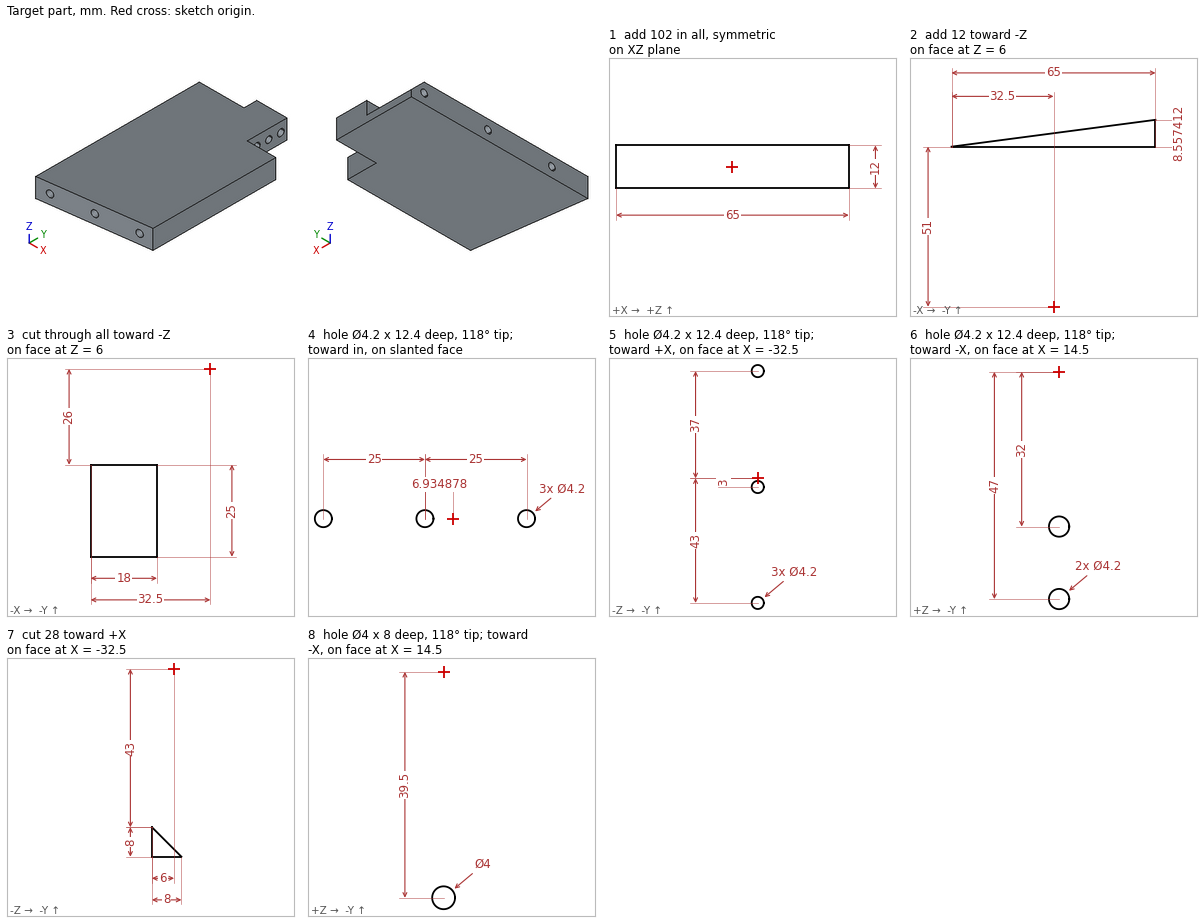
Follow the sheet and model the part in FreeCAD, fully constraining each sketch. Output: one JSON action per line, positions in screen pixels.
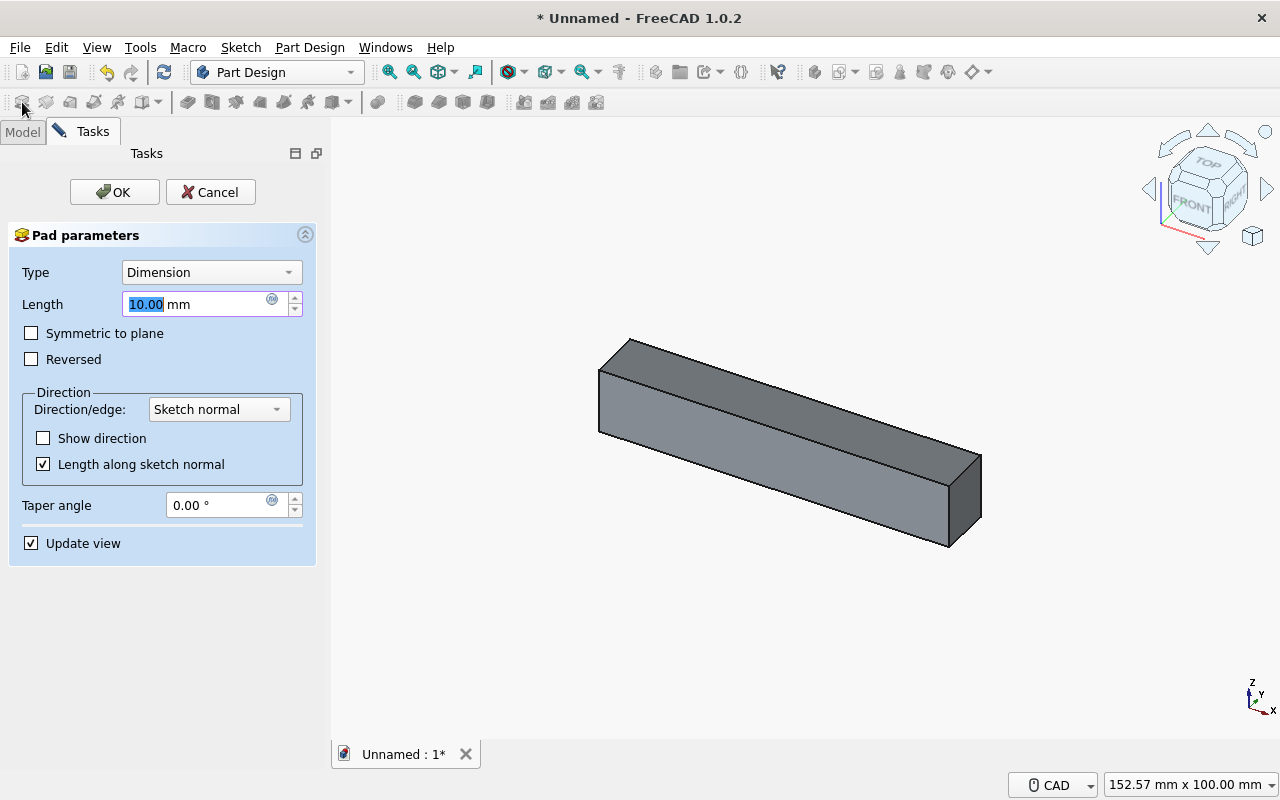
{"action": "type", "text": "102"}
{"action": "key", "text": "Tab"}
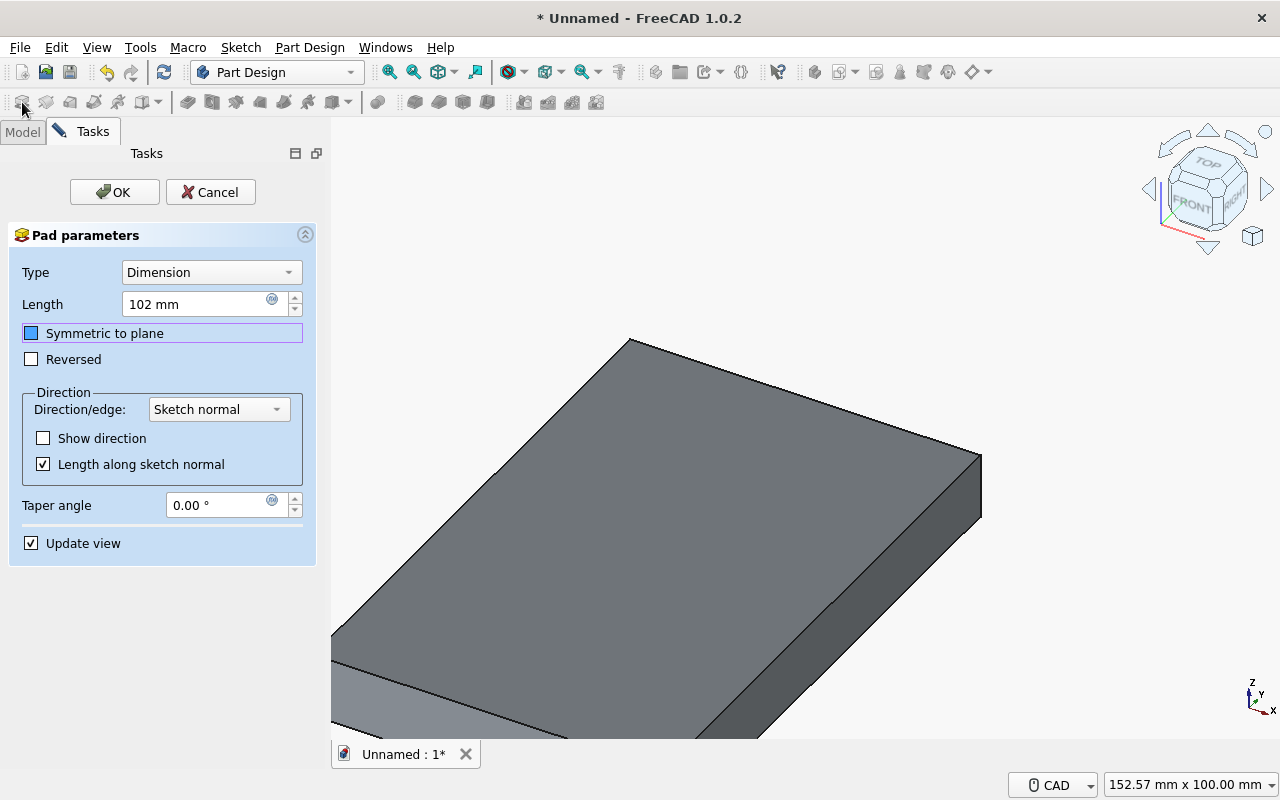
{"action": "left_click", "coordinate": [30, 333]}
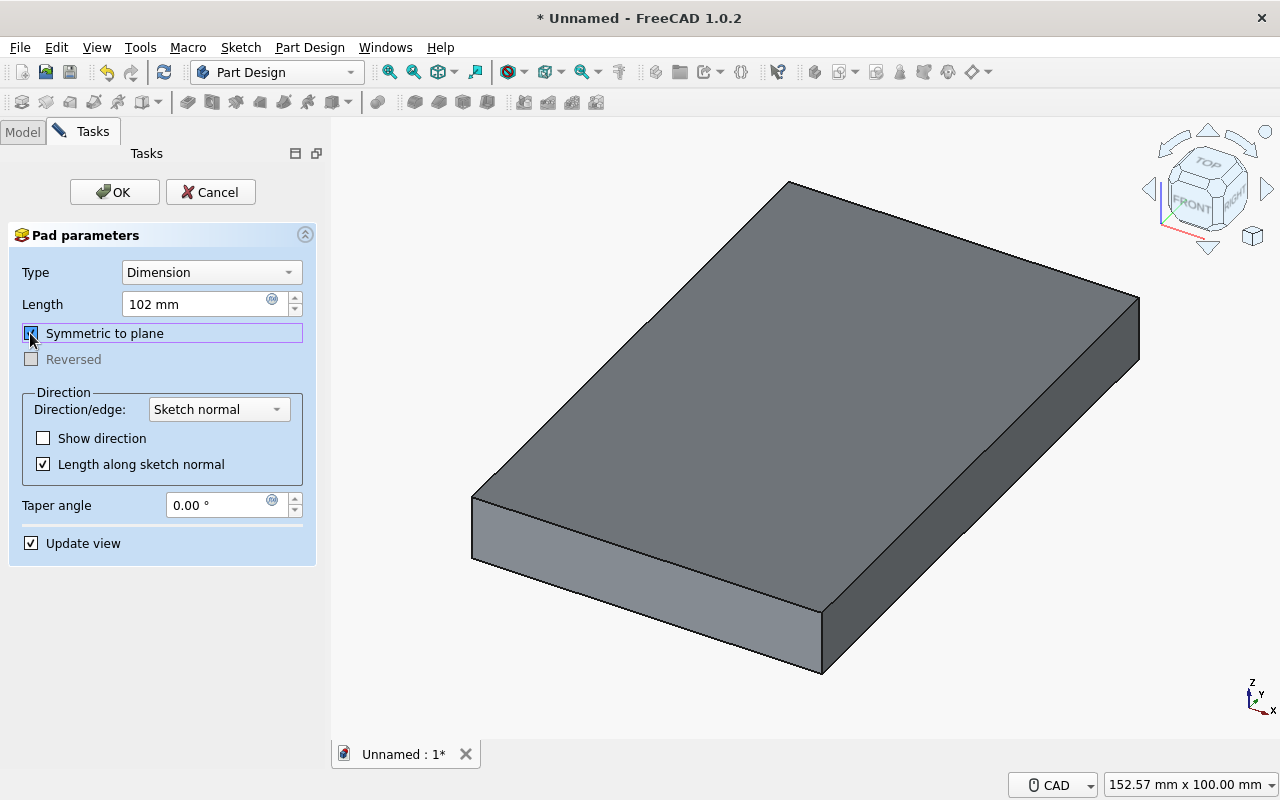
{"action": "left_click", "coordinate": [115, 192]}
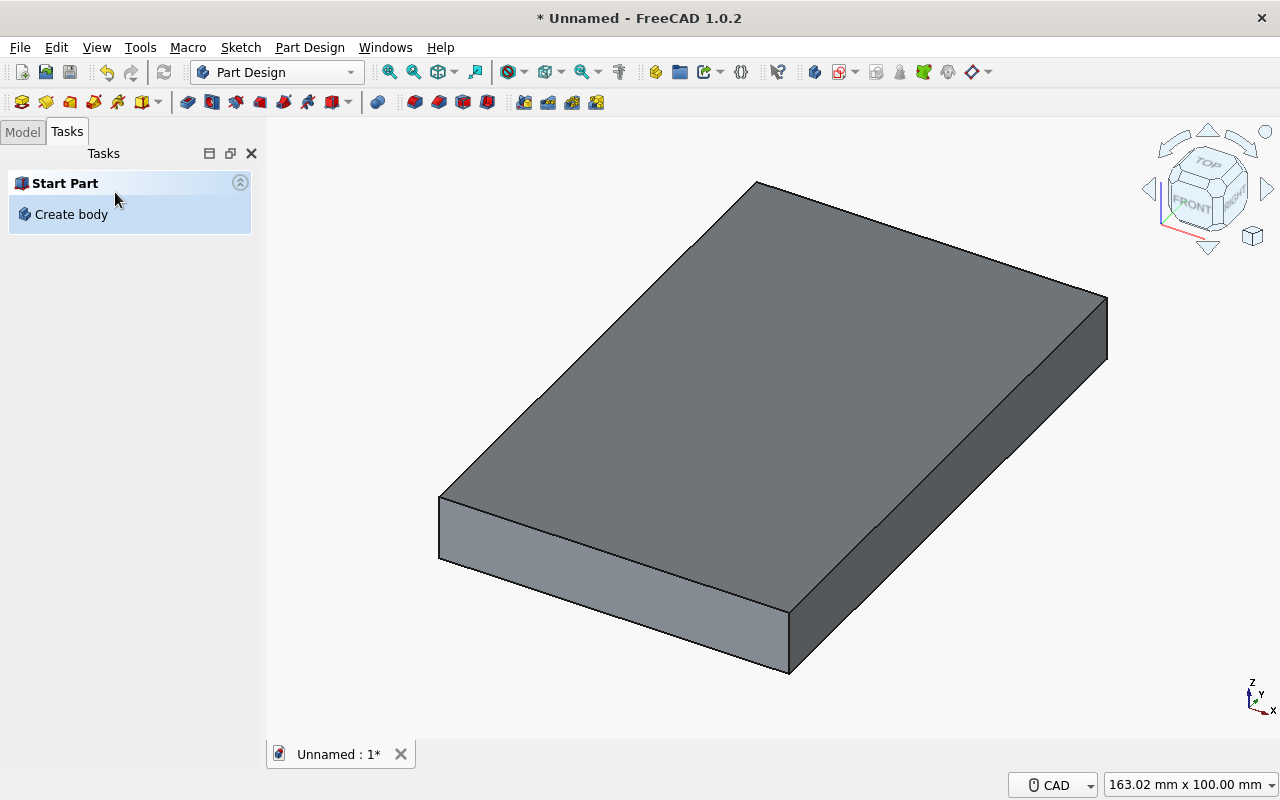
{"action": "left_click", "coordinate": [818, 351]}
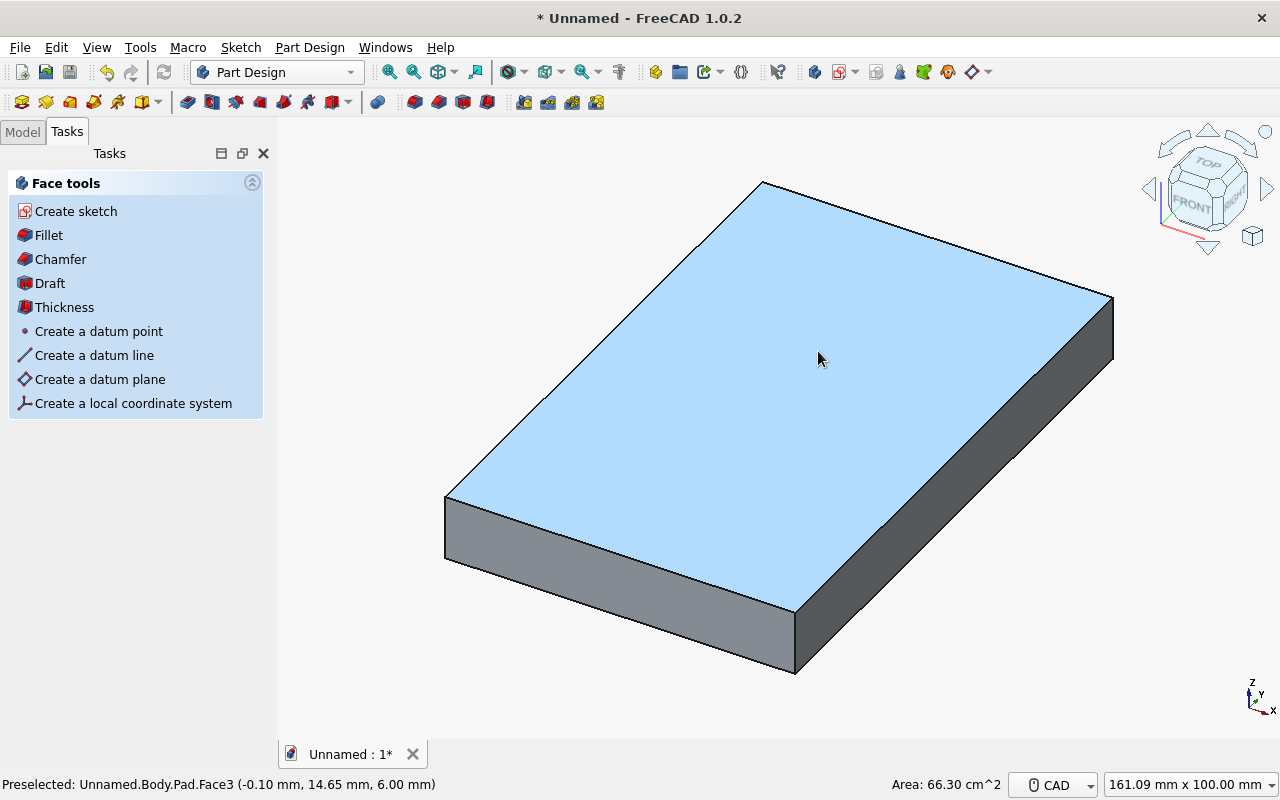
{"action": "left_click", "coordinate": [840, 72]}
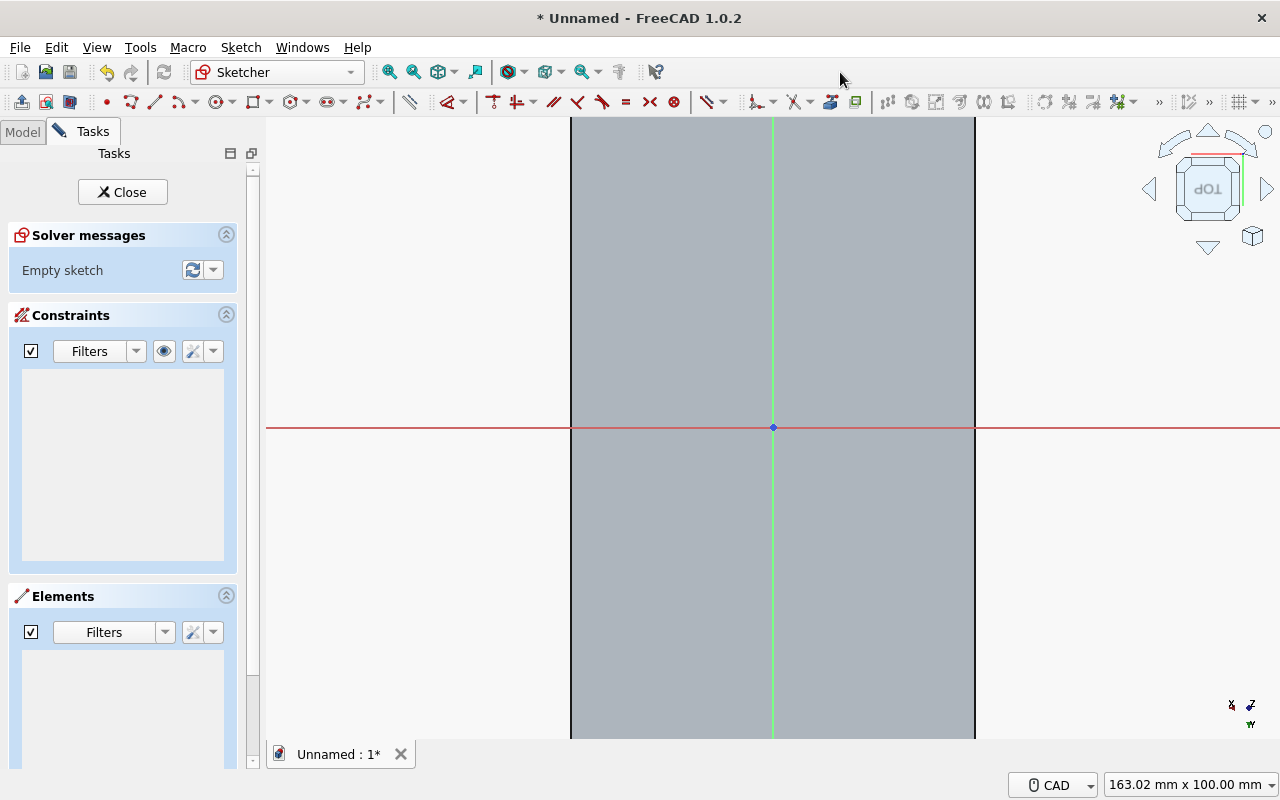
{"action": "scroll", "coordinate": [395, 711], "scroll_direction": "down", "scroll_amount": 1}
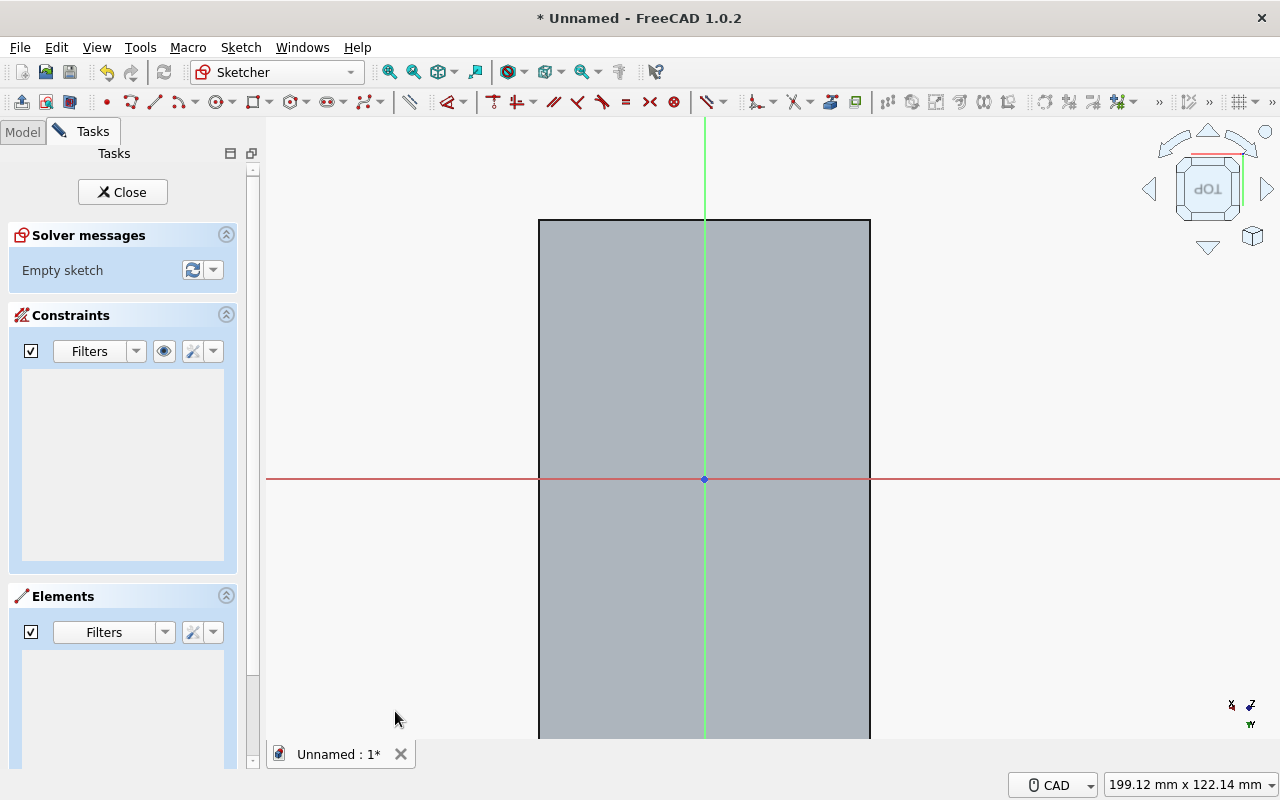
{"action": "key", "text": "g m"}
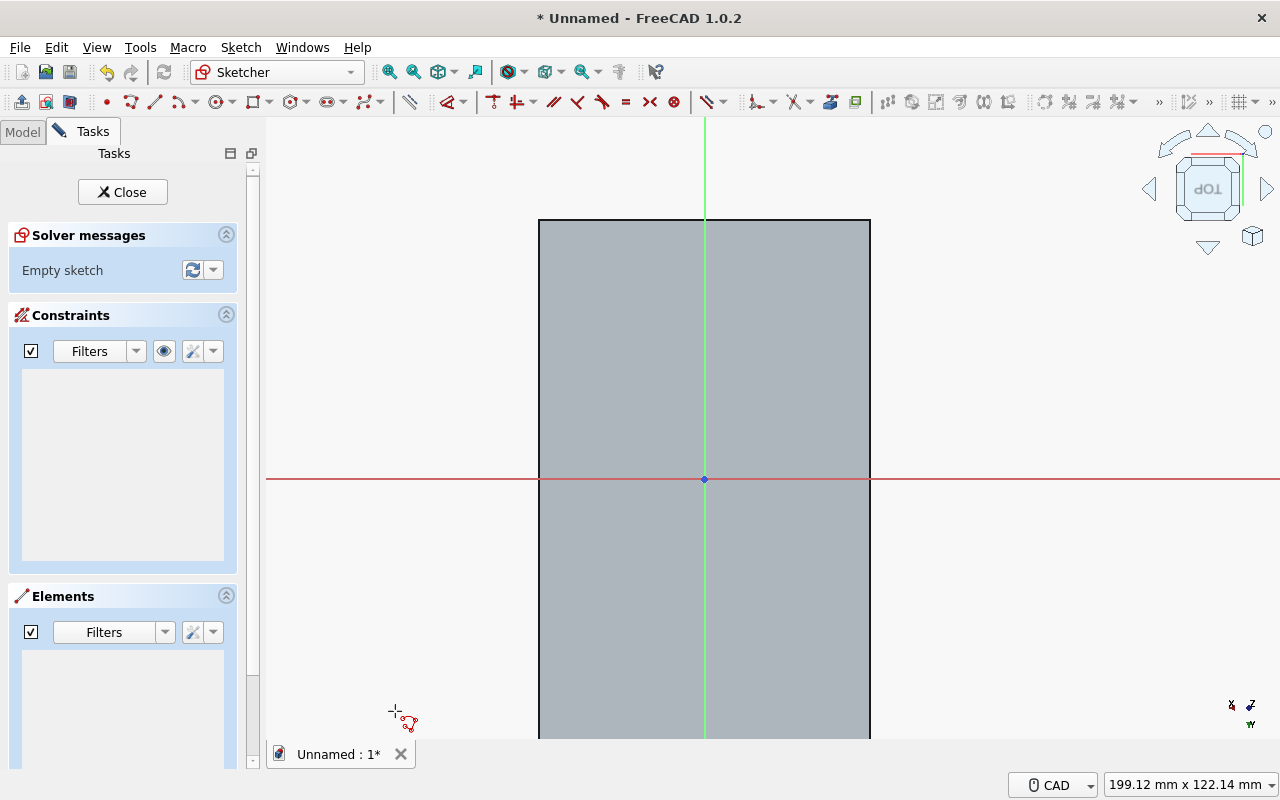
{"action": "left_click", "coordinate": [539, 220]}
{"action": "left_click", "coordinate": [870, 220]}
{"action": "left_click", "coordinate": [870, 176]}
{"action": "left_click", "coordinate": [539, 221]}
{"action": "key", "text": "Escape"}
{"action": "key", "text": "Escape"}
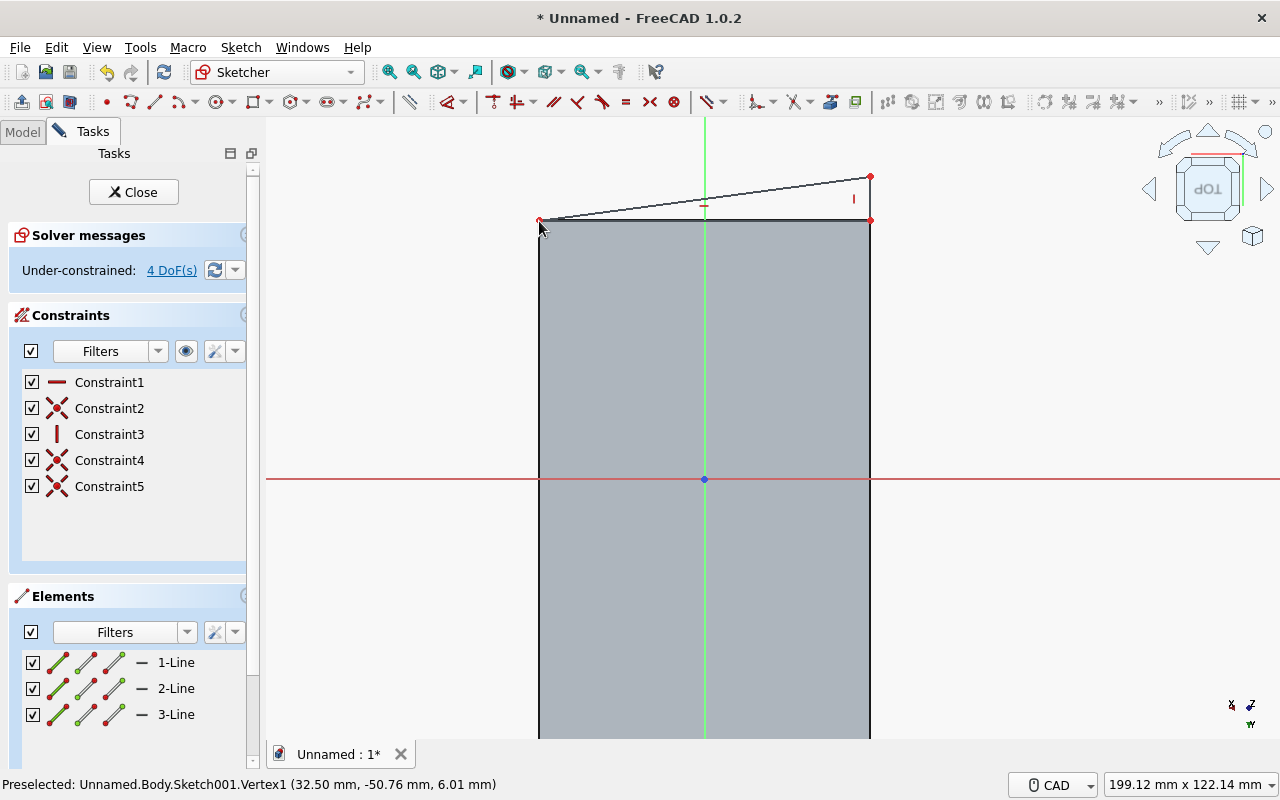
{"action": "left_click", "coordinate": [448, 102]}